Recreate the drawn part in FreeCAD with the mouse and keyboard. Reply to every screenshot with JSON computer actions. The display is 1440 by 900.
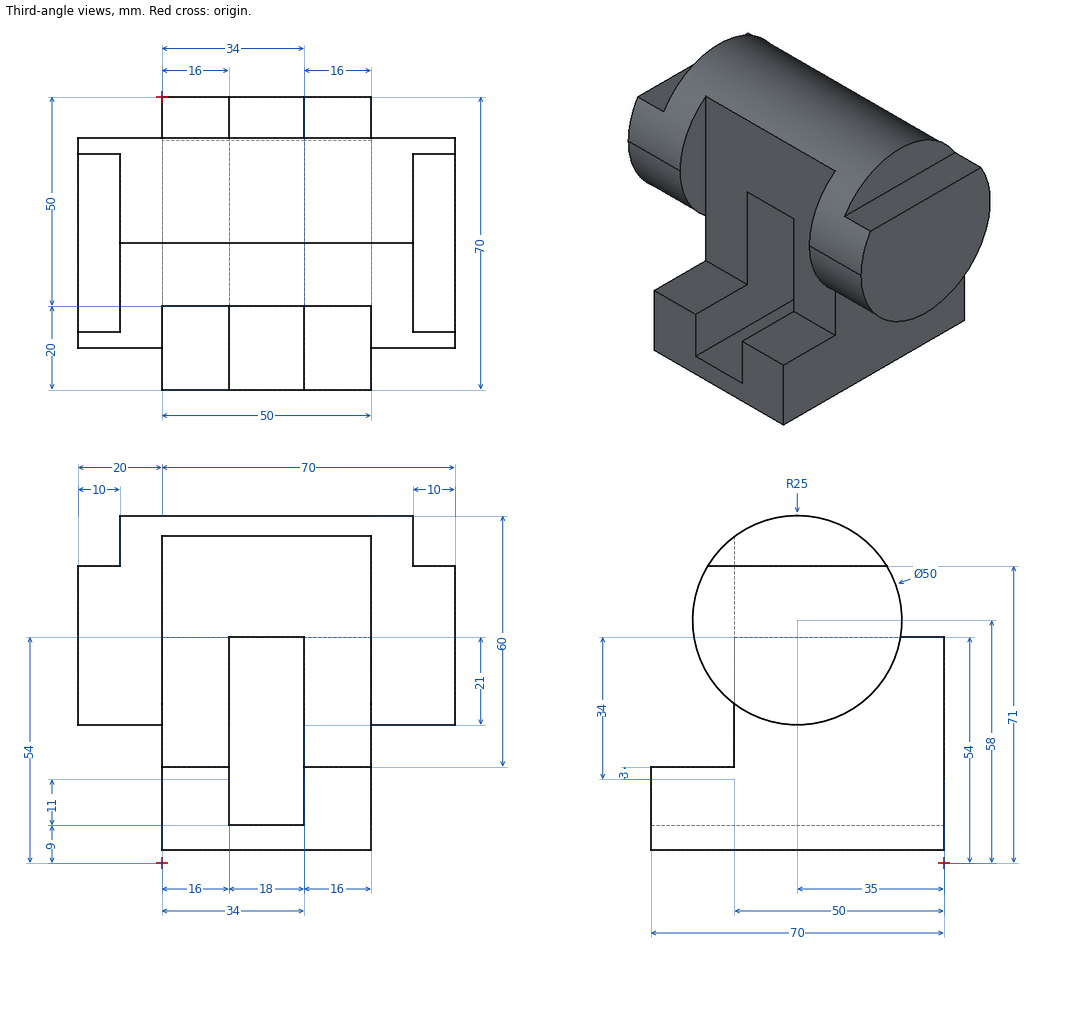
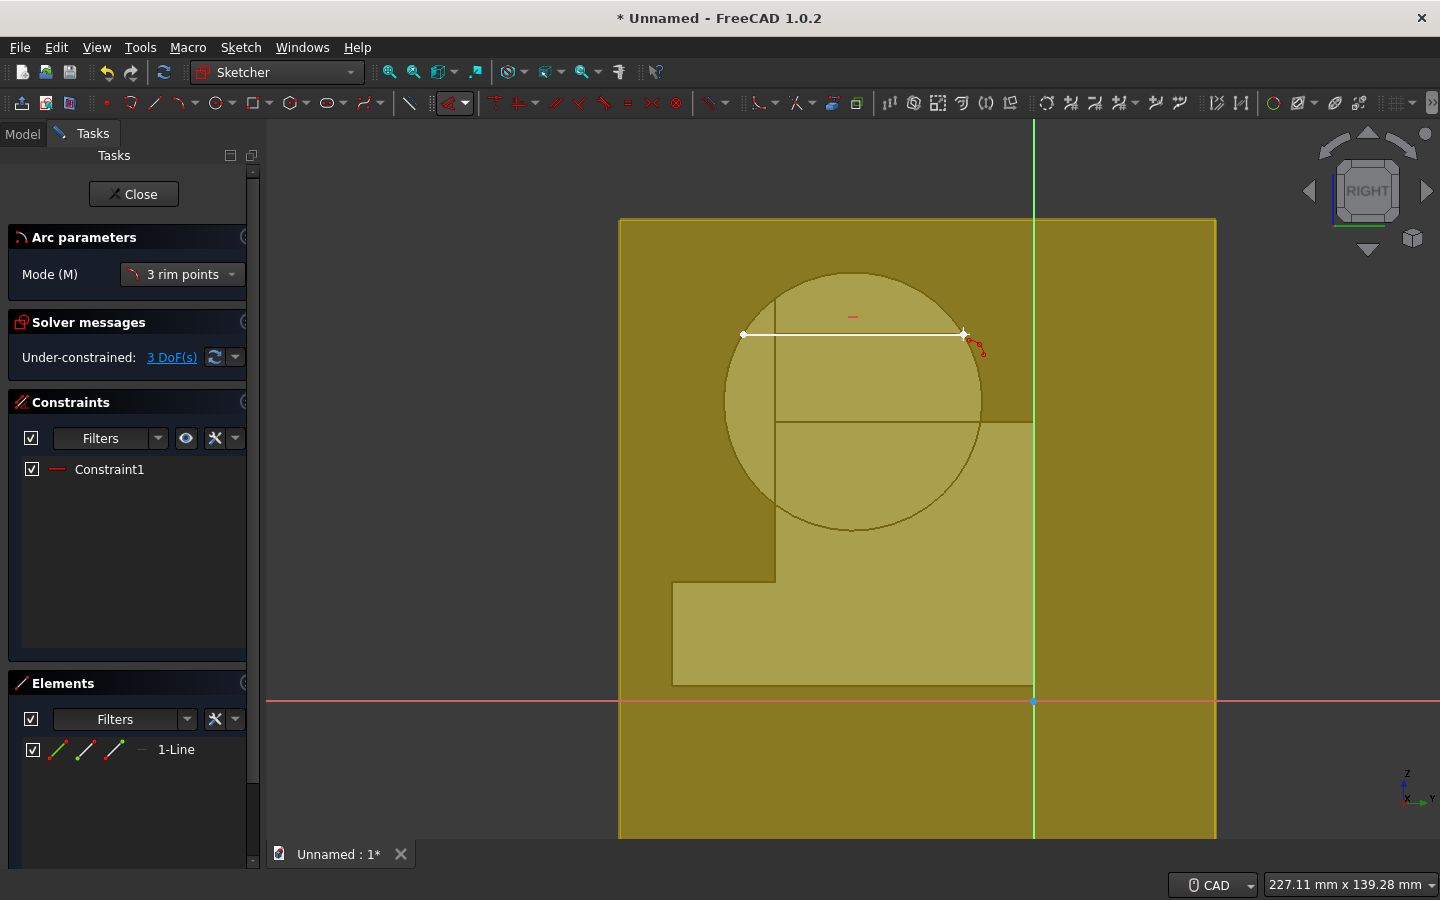
{"action": "left_click", "coordinate": [963, 335]}
{"action": "left_click", "coordinate": [743, 335]}
{"action": "left_click", "coordinate": [853, 272]}
{"action": "key", "text": "Escape"}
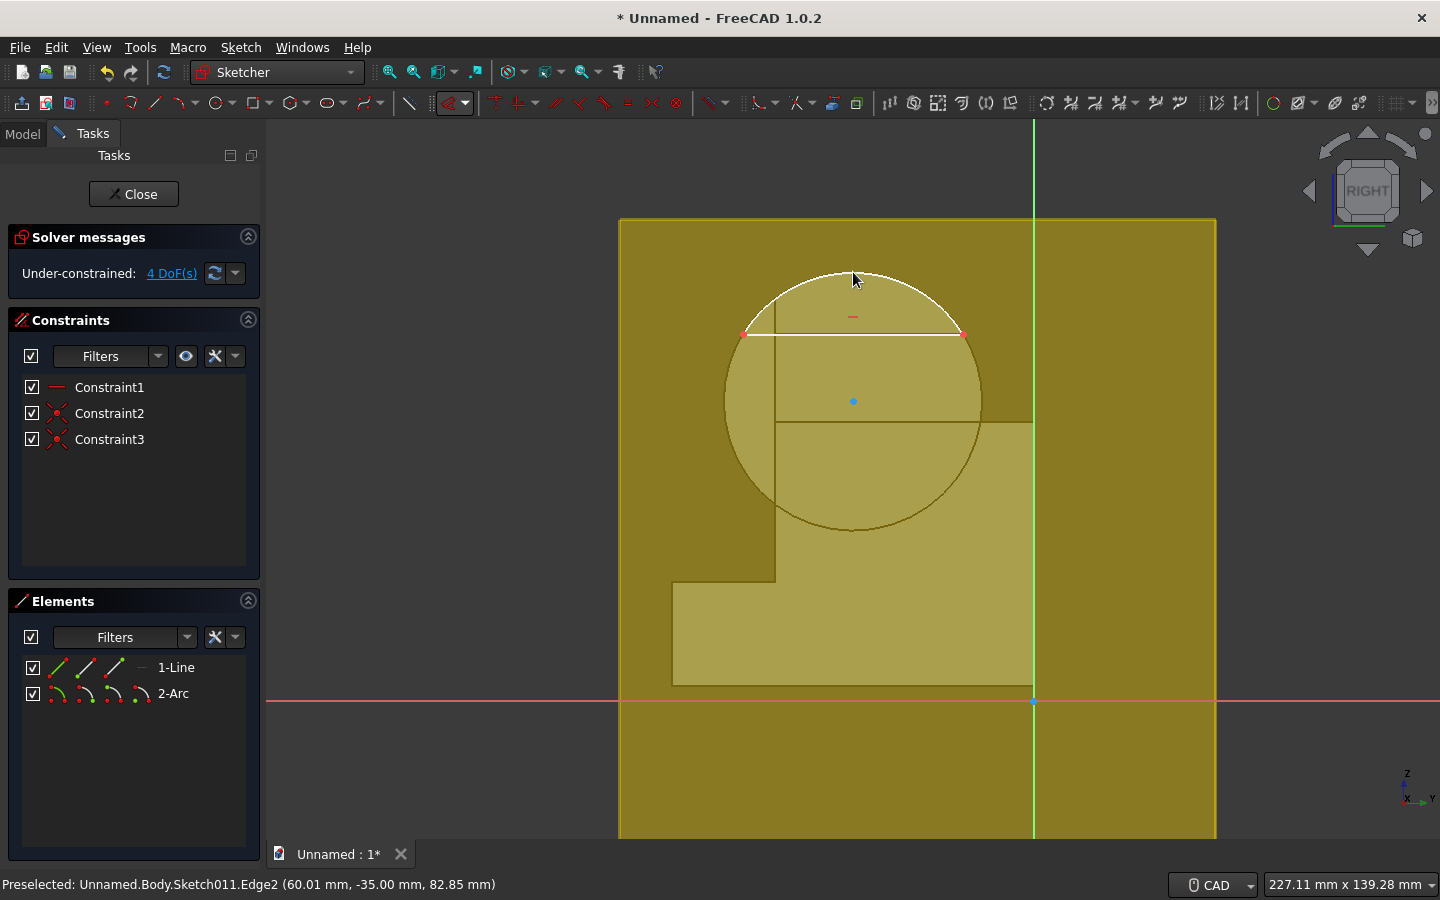
{"action": "left_click", "coordinate": [904, 284]}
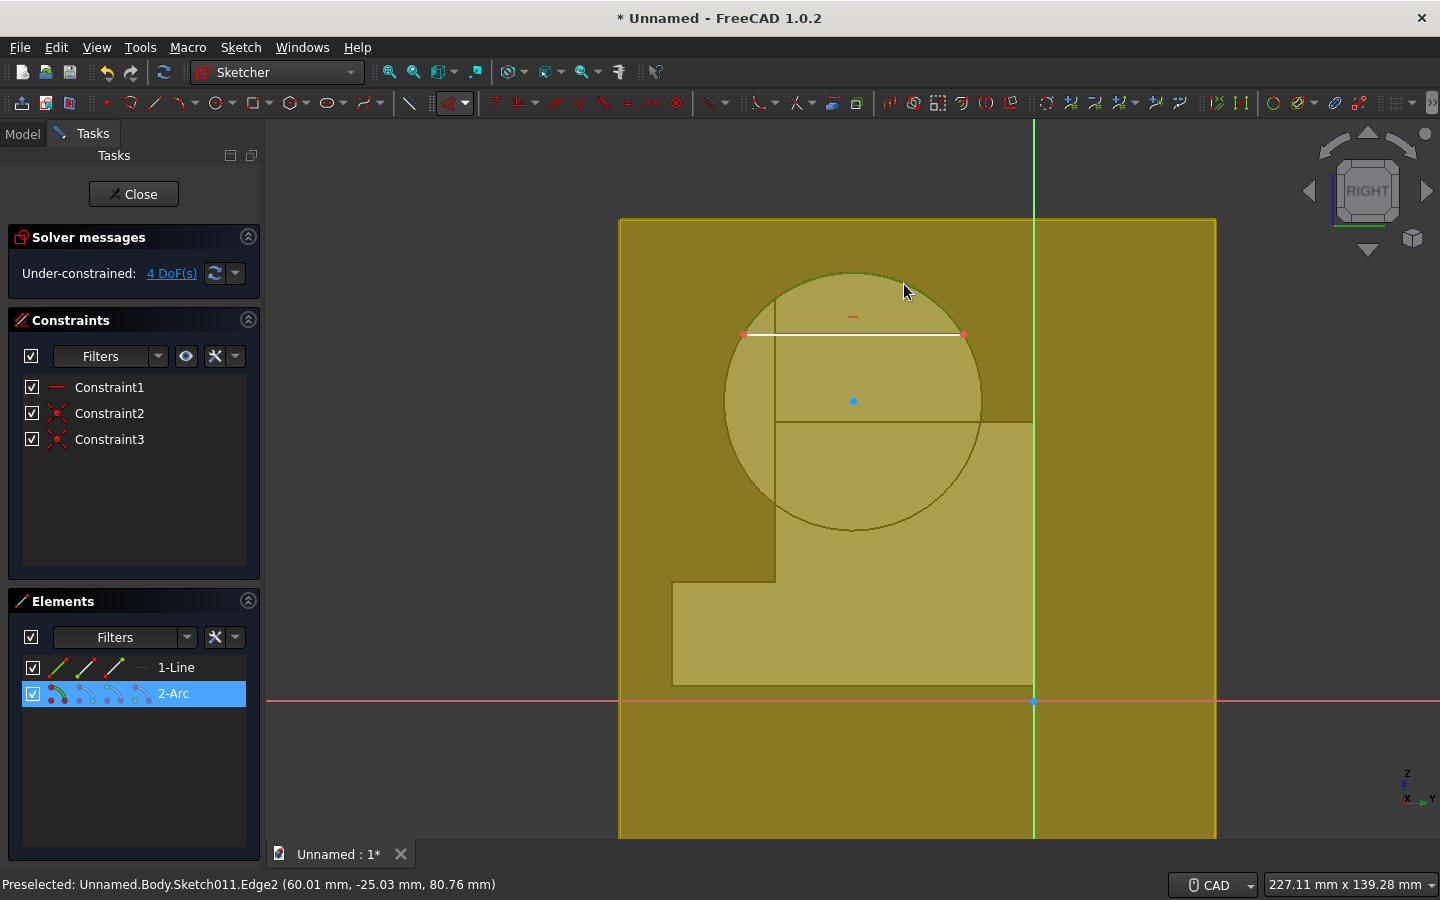
{"action": "key", "text": "k r"}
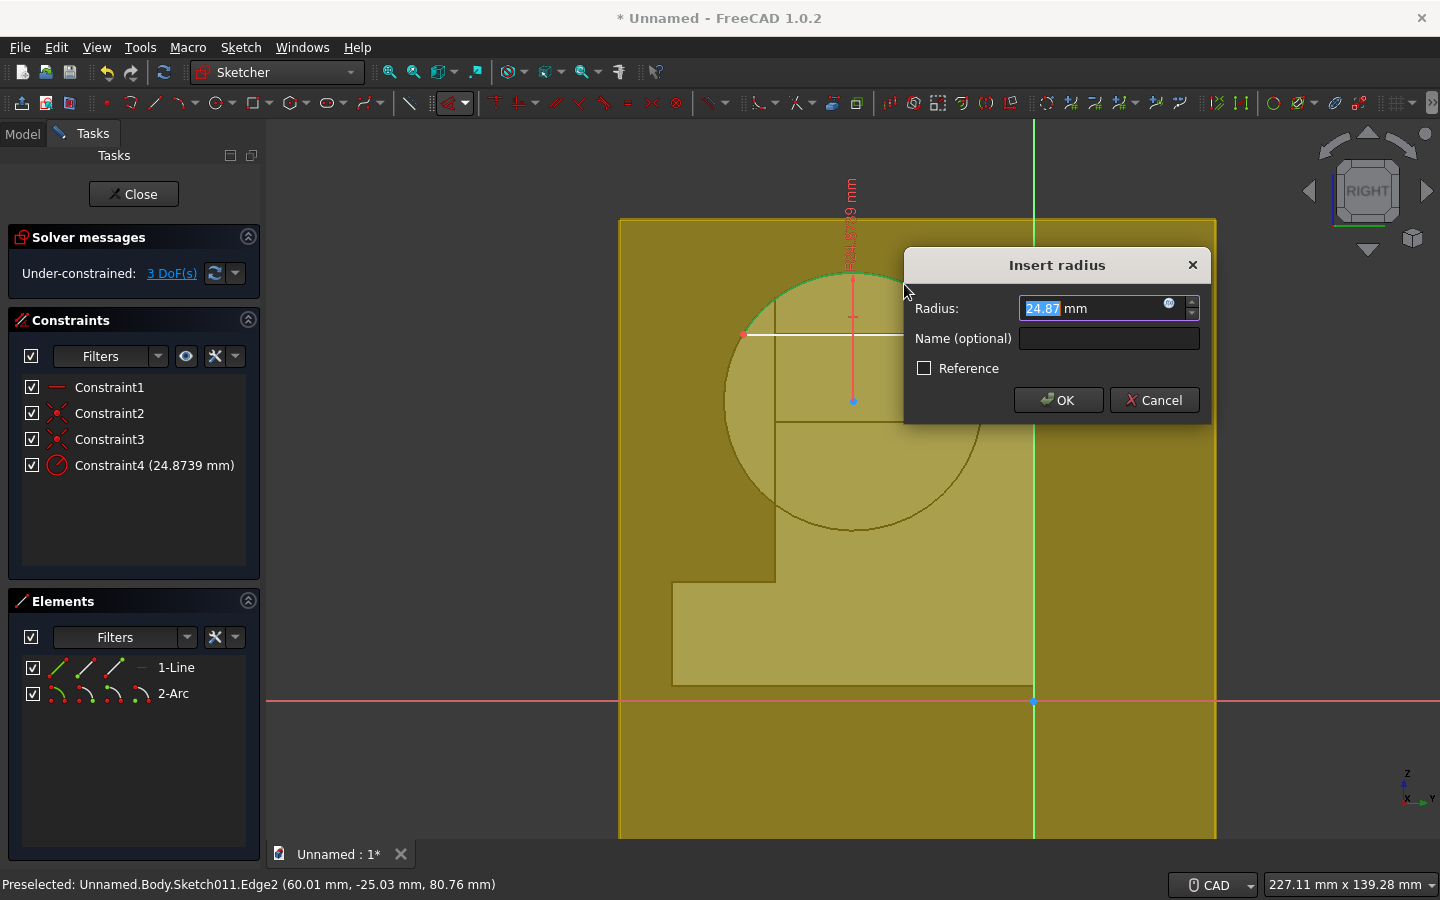
{"action": "type", "text": "25"}
{"action": "key", "text": "Return"}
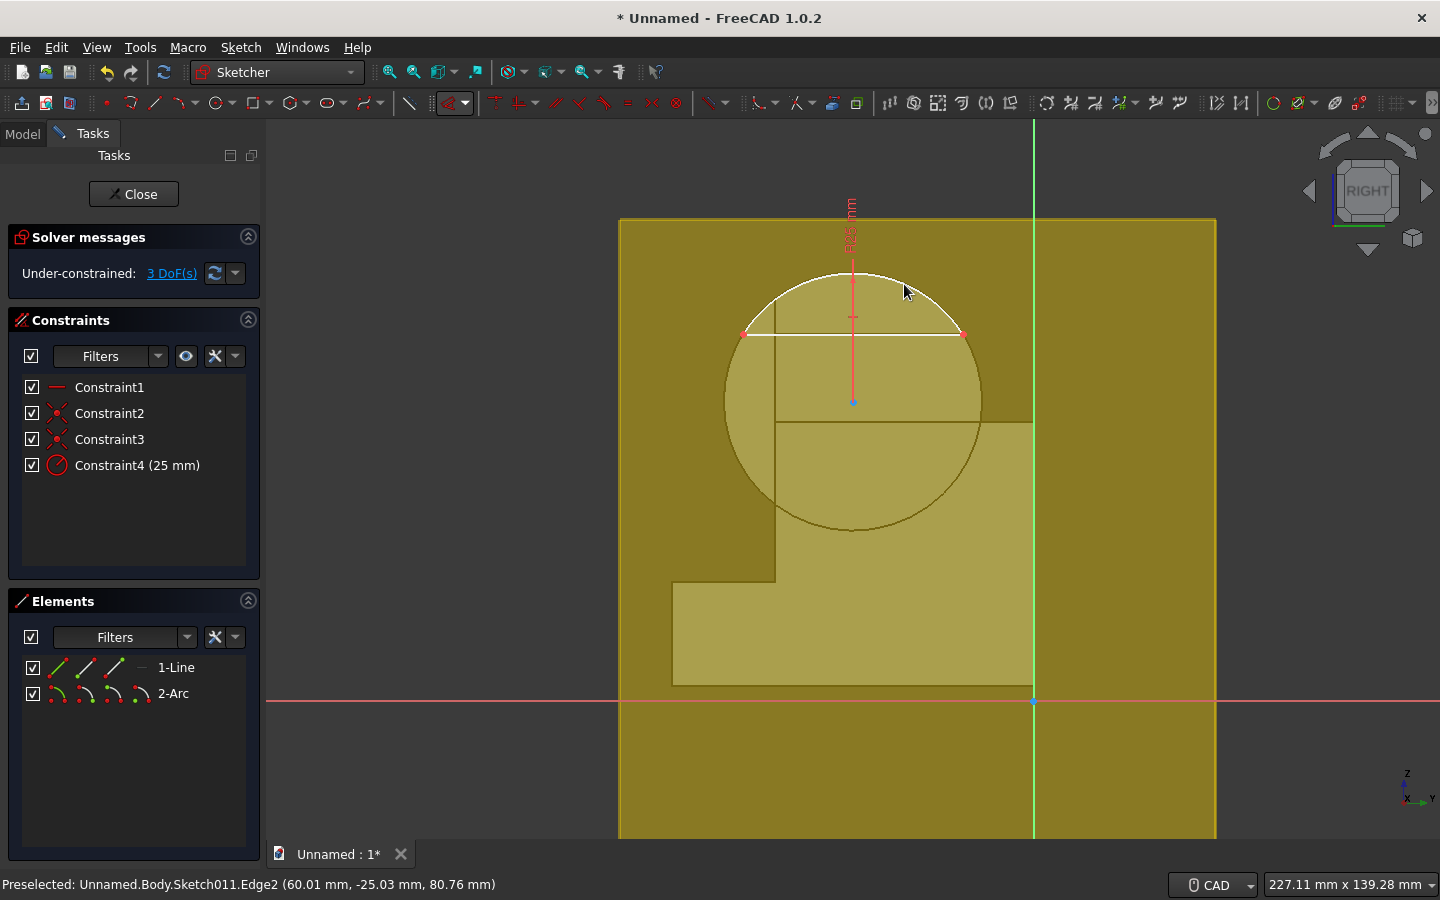
{"action": "left_click", "coordinate": [743, 335]}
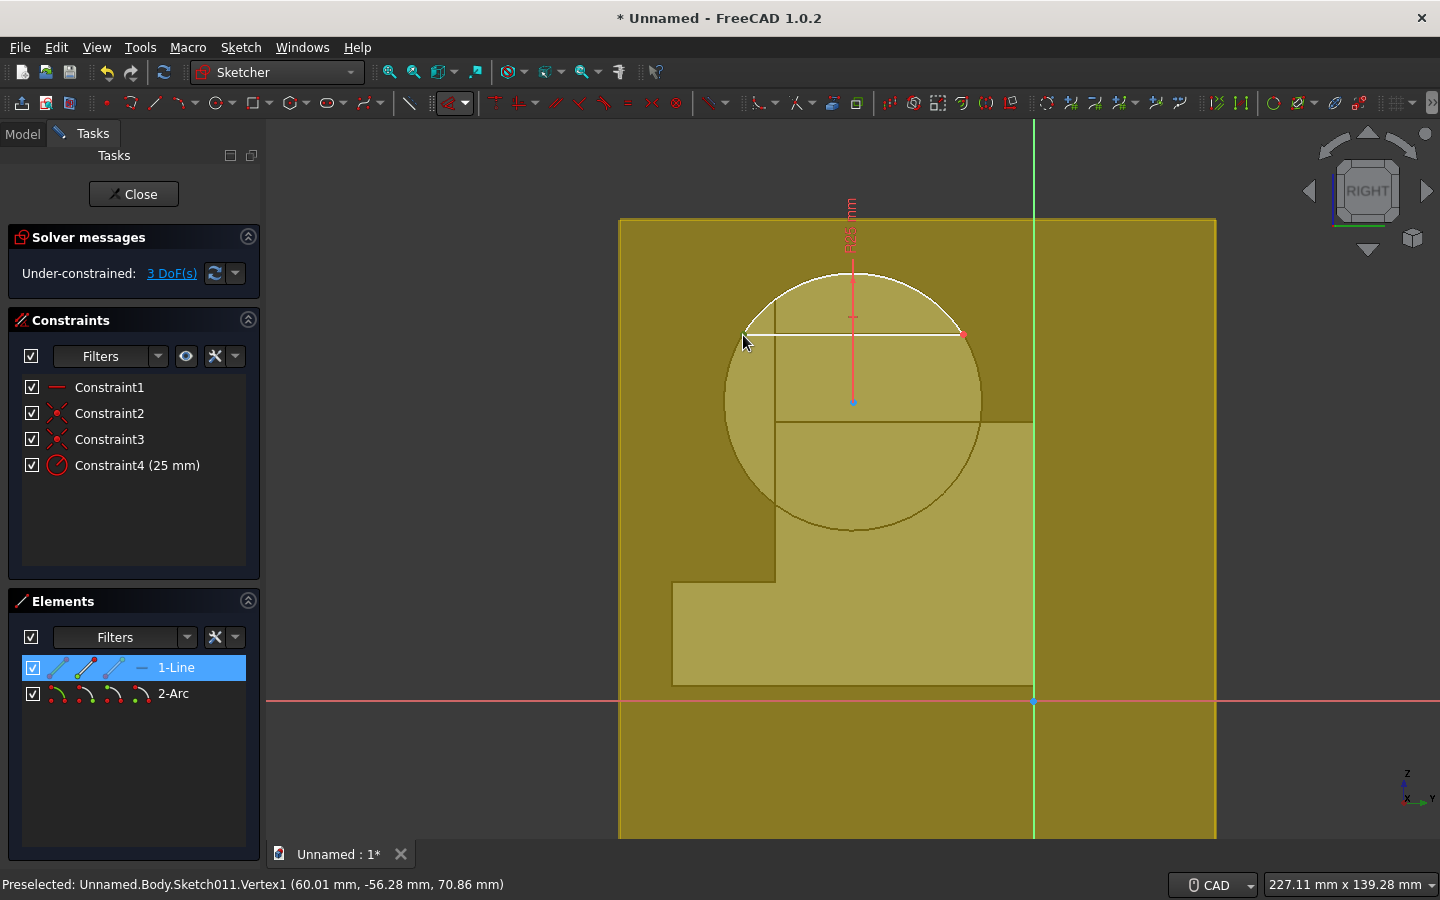
{"action": "left_click", "coordinate": [468, 104]}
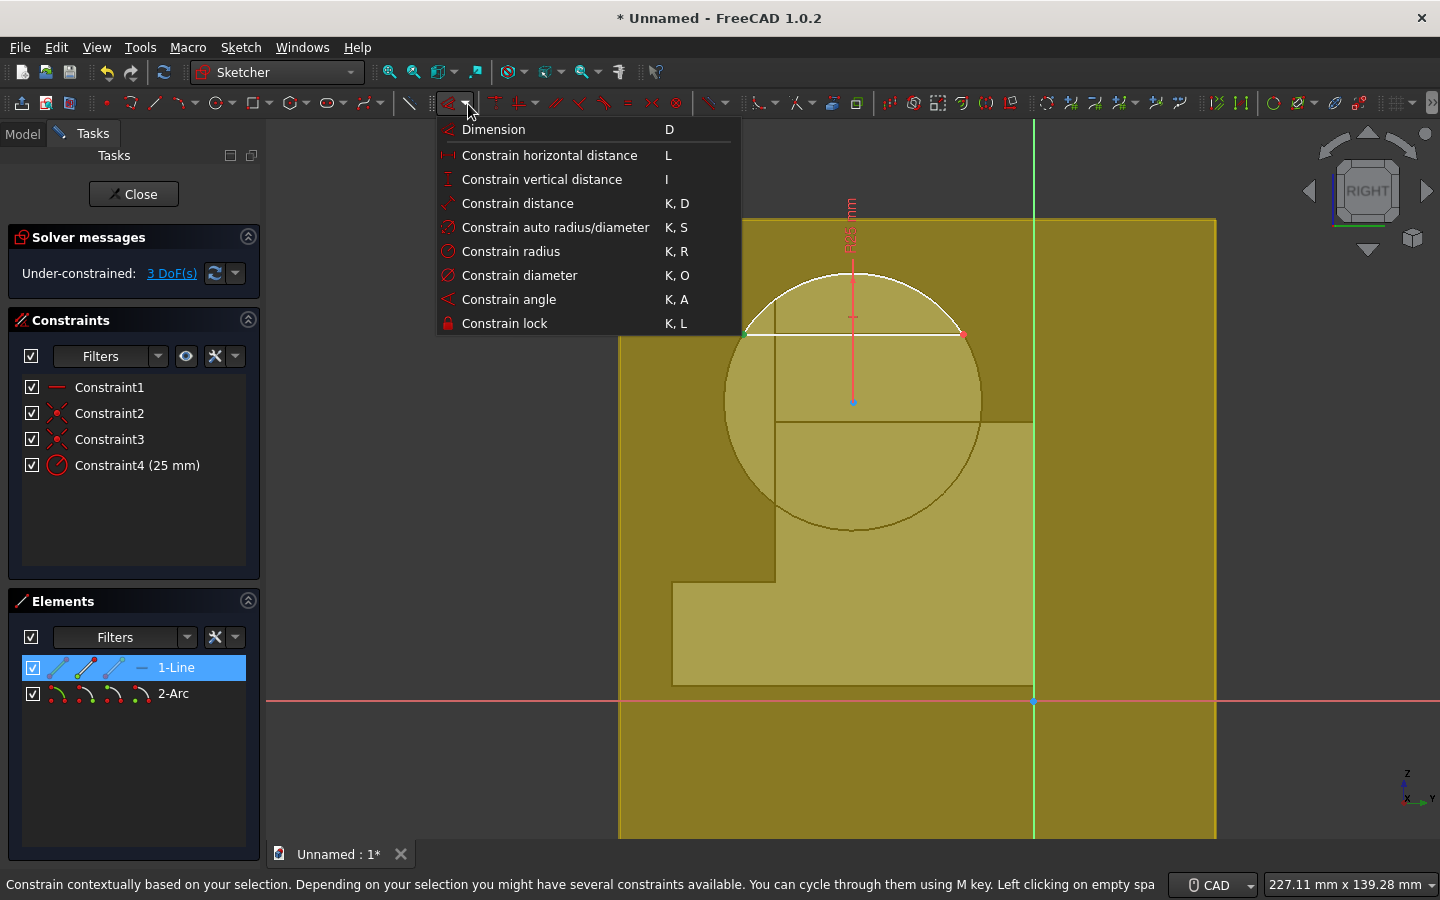
{"action": "left_click", "coordinate": [589, 179]}